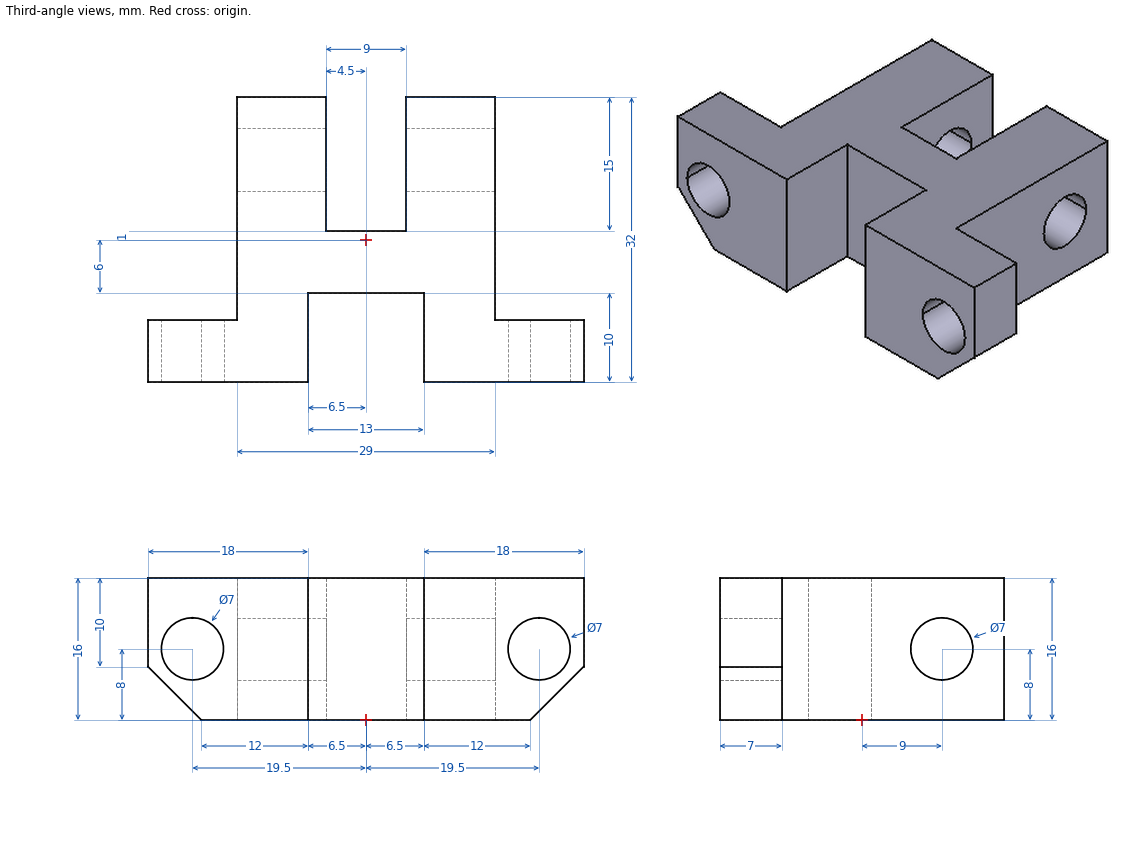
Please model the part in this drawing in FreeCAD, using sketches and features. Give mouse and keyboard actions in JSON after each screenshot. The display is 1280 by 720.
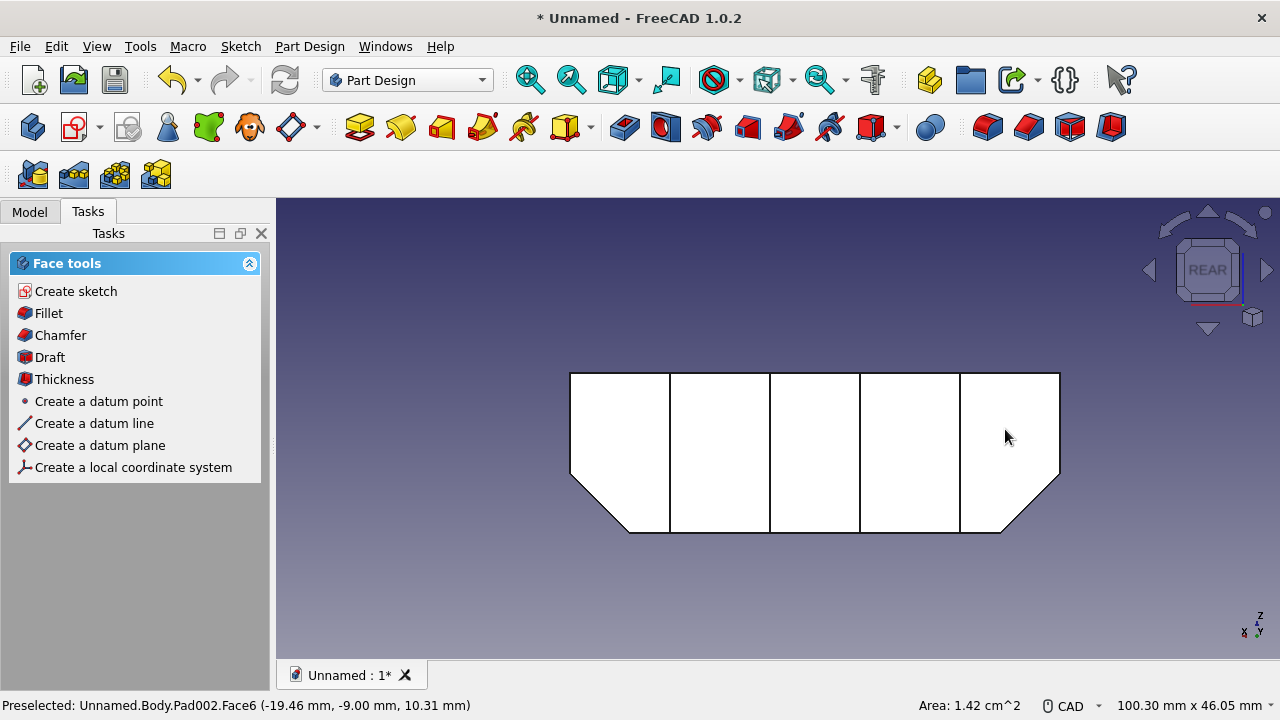
{"action": "left_click", "coordinate": [74, 128]}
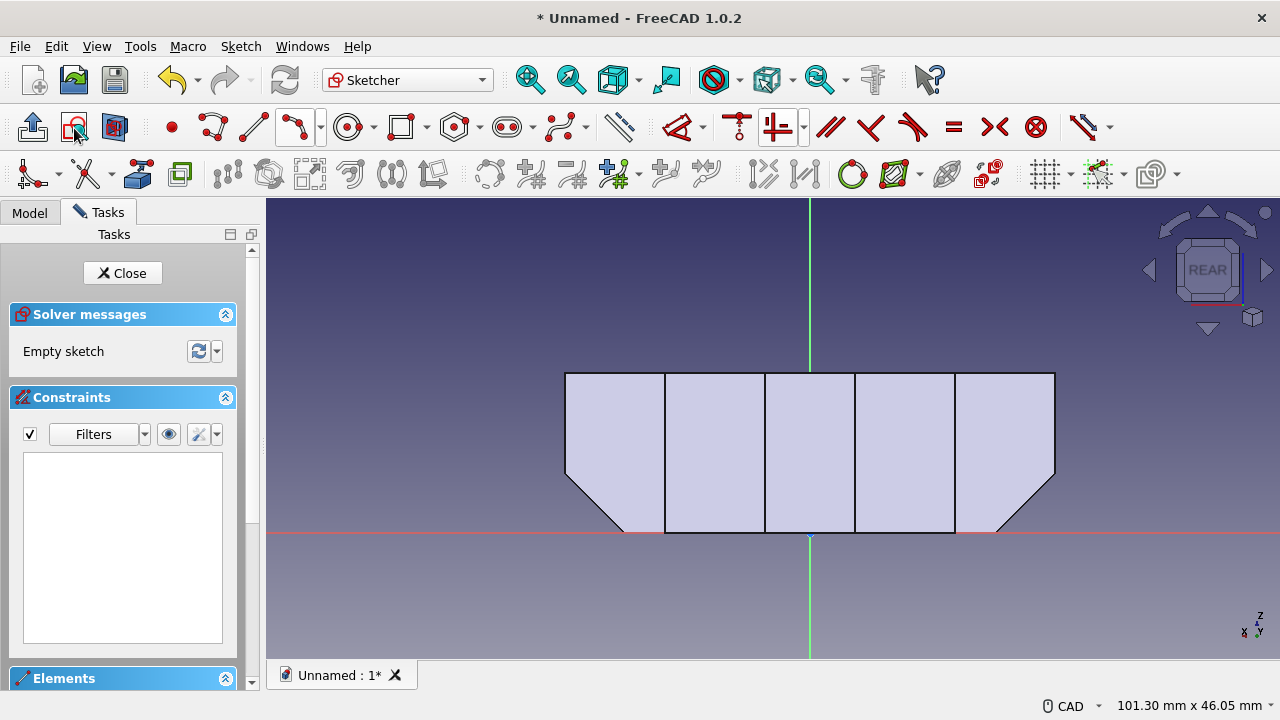
{"action": "left_click", "coordinate": [115, 128]}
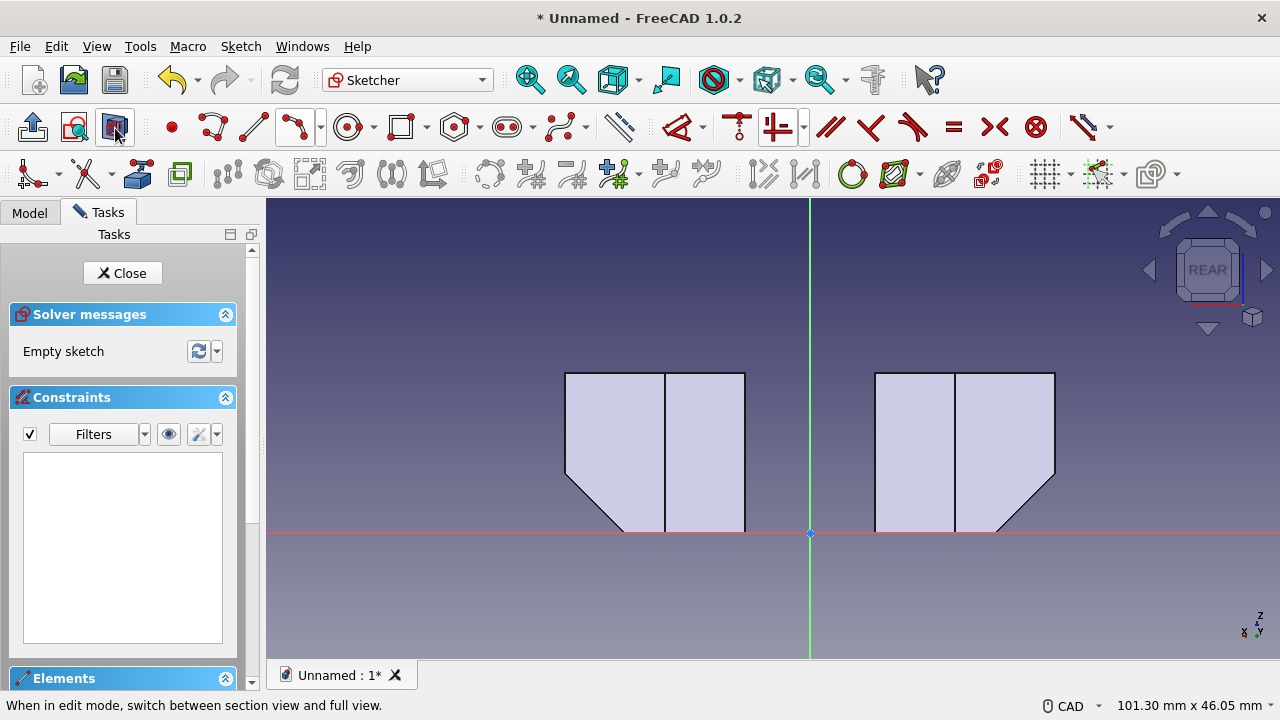
{"action": "scroll", "coordinate": [1104, 461], "scroll_direction": "up", "scroll_amount": 7}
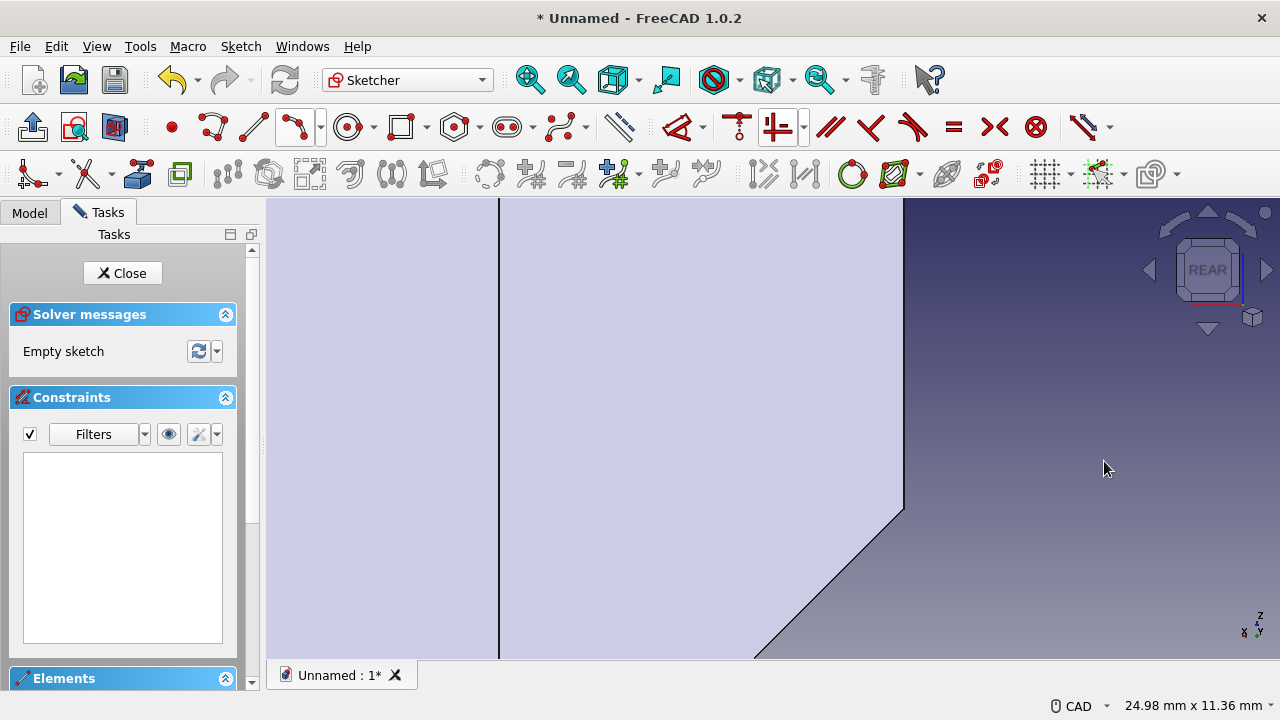
{"action": "left_click", "coordinate": [348, 128]}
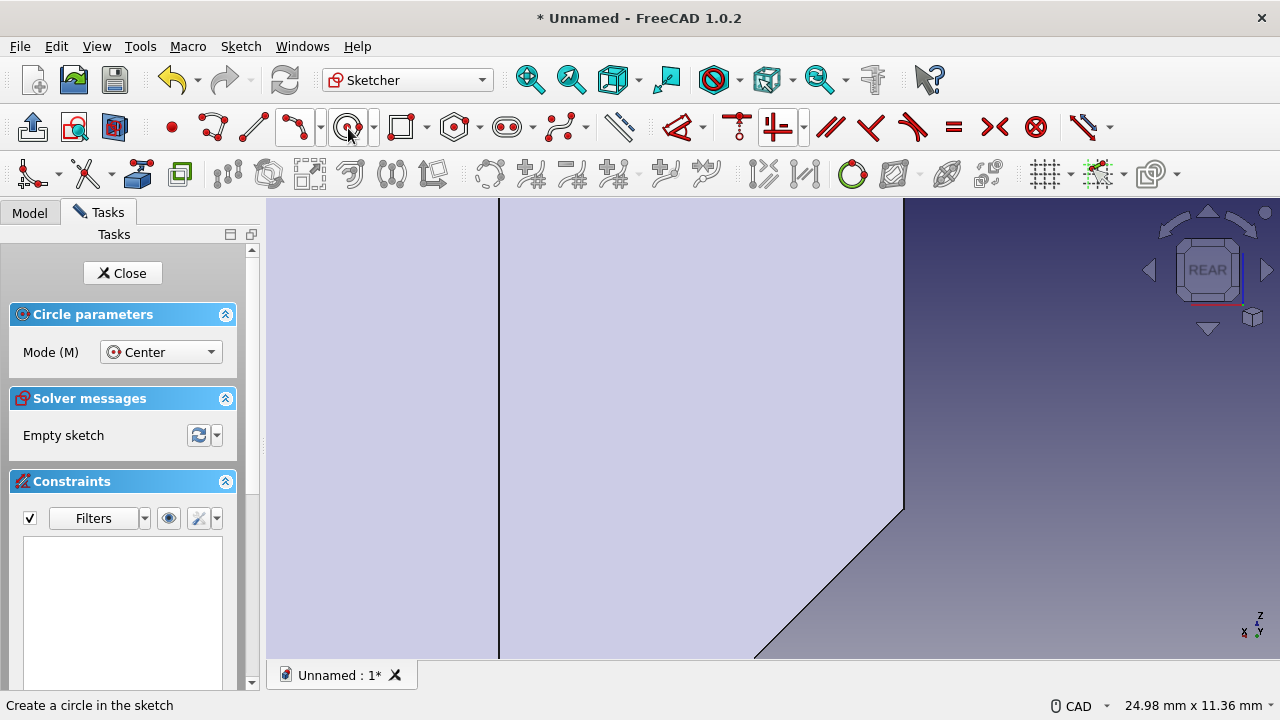
{"action": "left_click", "coordinate": [701, 427]}
{"action": "mouse_move", "coordinate": [802, 327]}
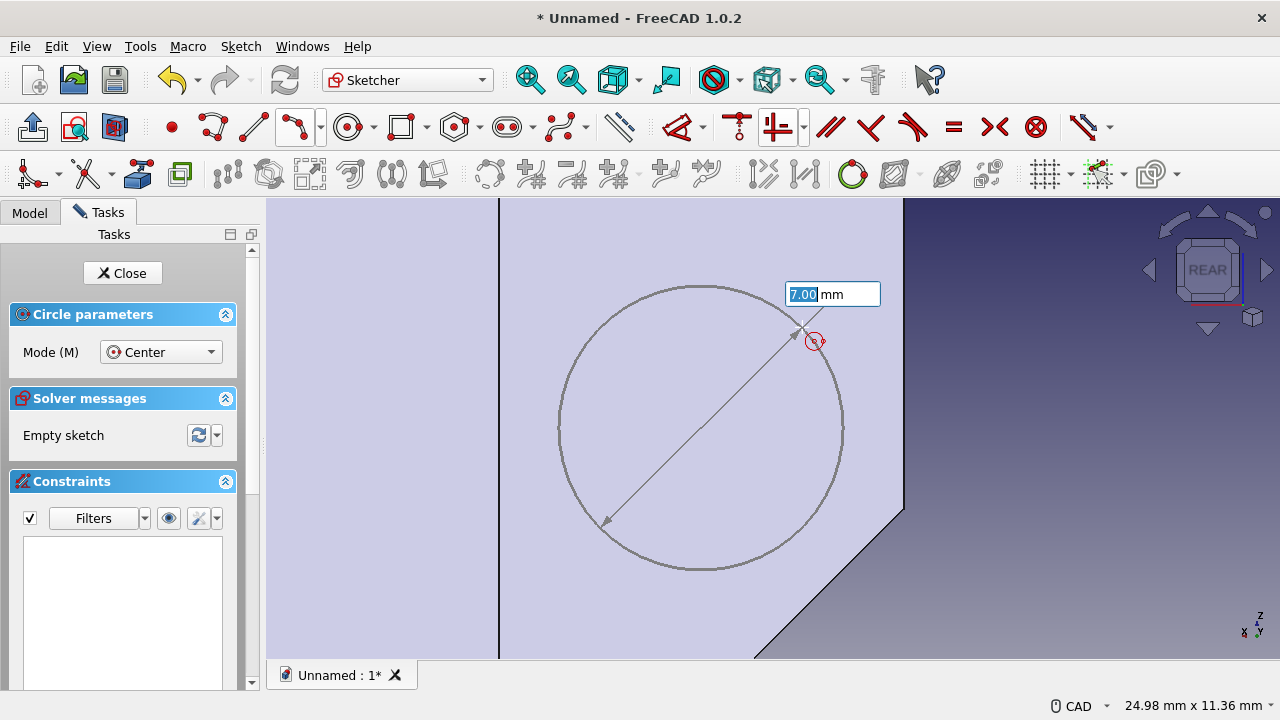
{"action": "type", "text": "7"}
{"action": "key", "text": "Return"}
{"action": "key", "text": "Escape"}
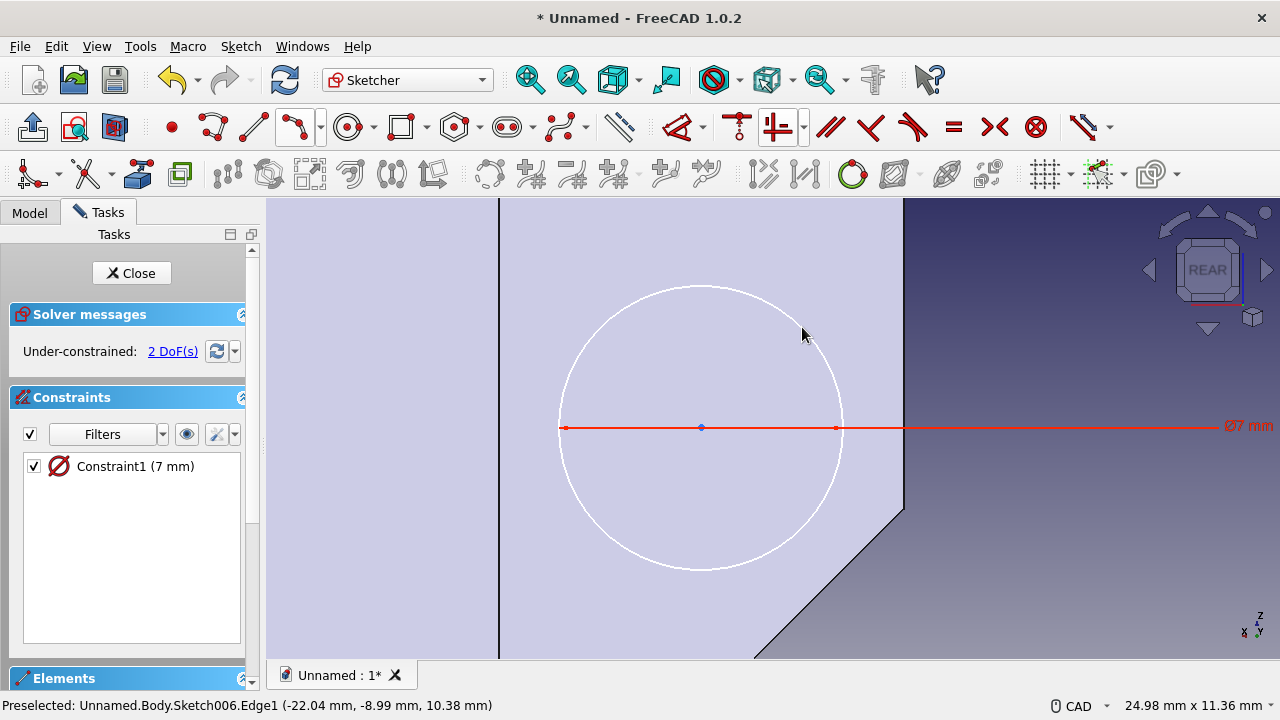
{"action": "left_click", "coordinate": [676, 128]}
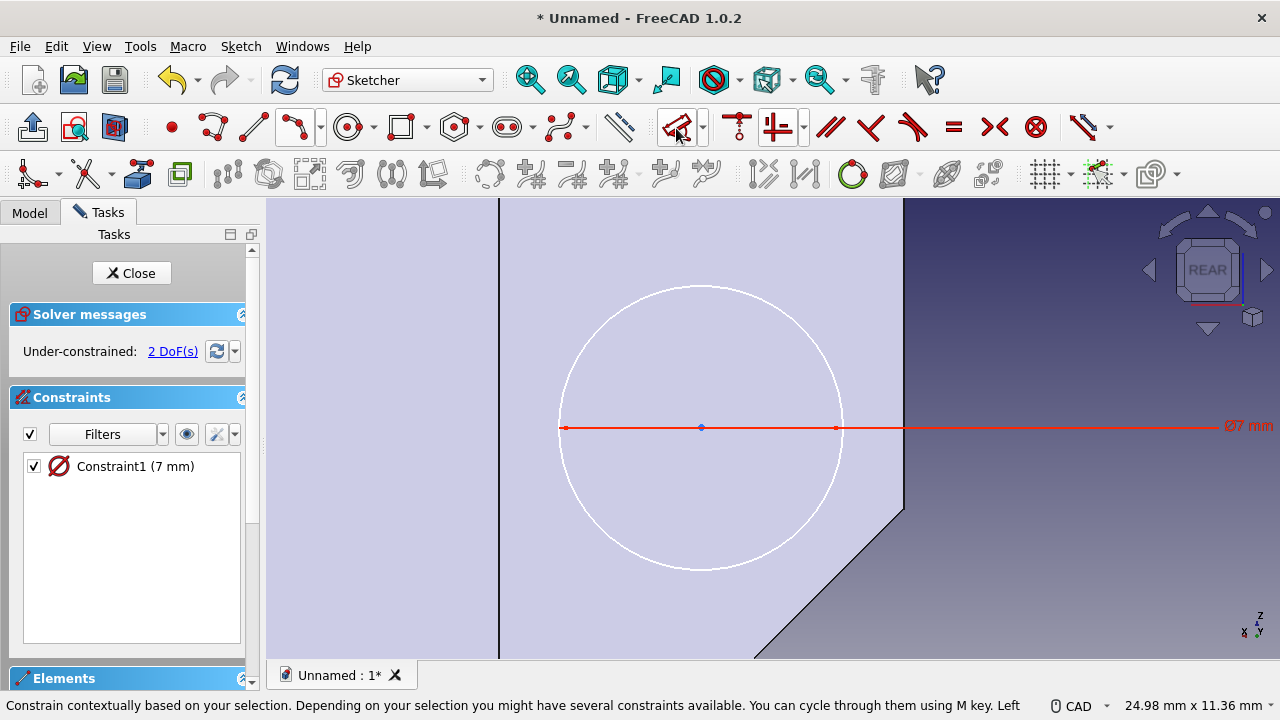
{"action": "left_click", "coordinate": [701, 428]}
{"action": "left_click", "coordinate": [735, 529]}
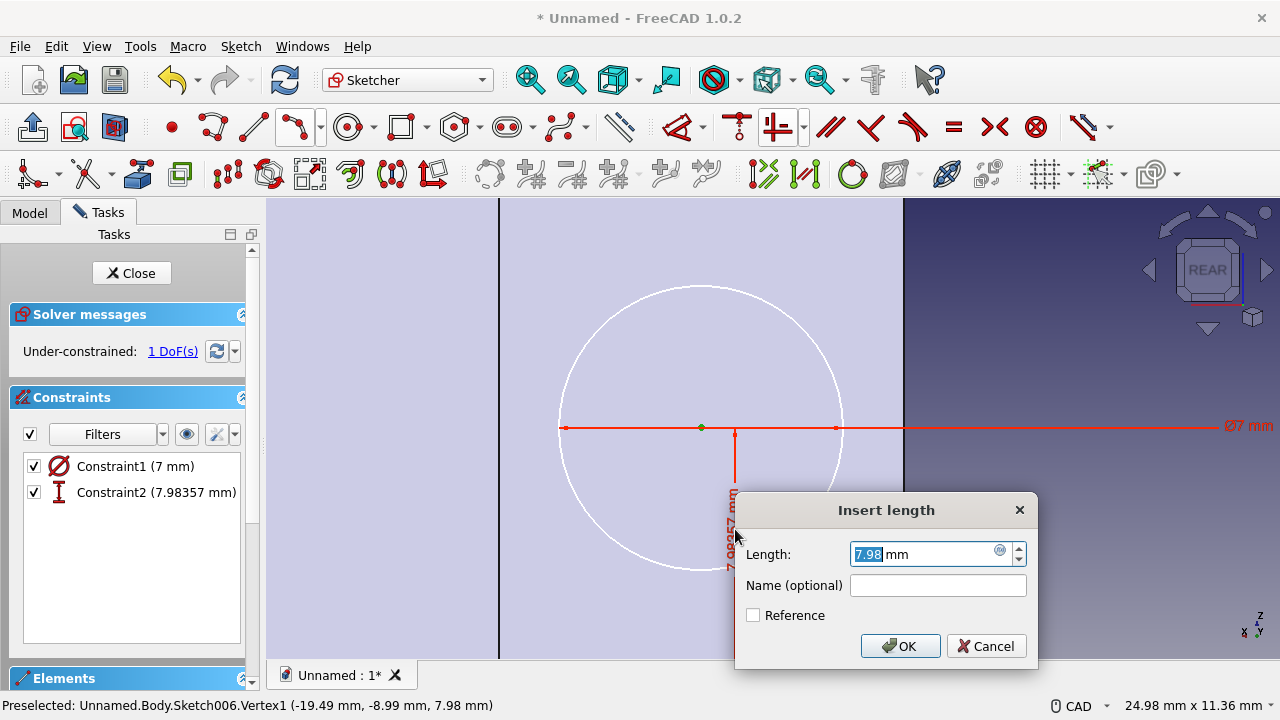
{"action": "type", "text": "8"}
{"action": "key", "text": "Return"}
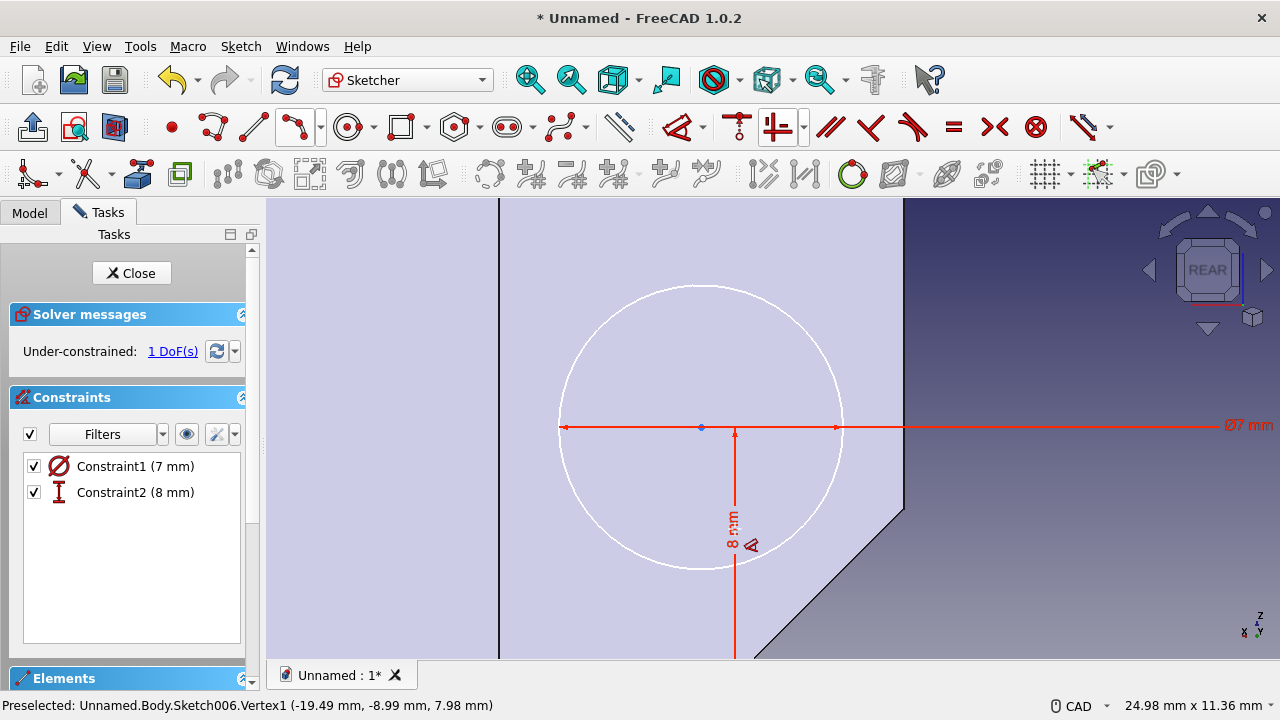
{"action": "left_click", "coordinate": [701, 427]}
{"action": "left_click", "coordinate": [498, 393]}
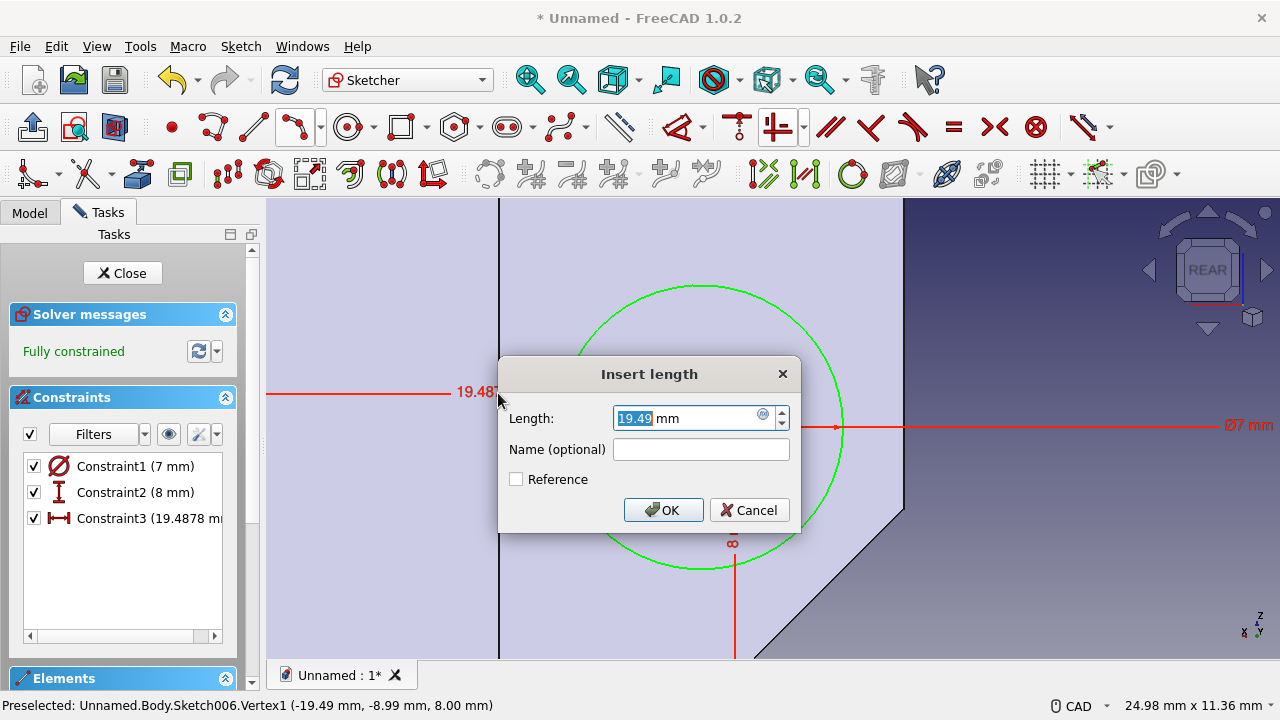
{"action": "type", "text": "19.5"}
{"action": "key", "text": "Return"}
{"action": "key", "text": "Escape"}